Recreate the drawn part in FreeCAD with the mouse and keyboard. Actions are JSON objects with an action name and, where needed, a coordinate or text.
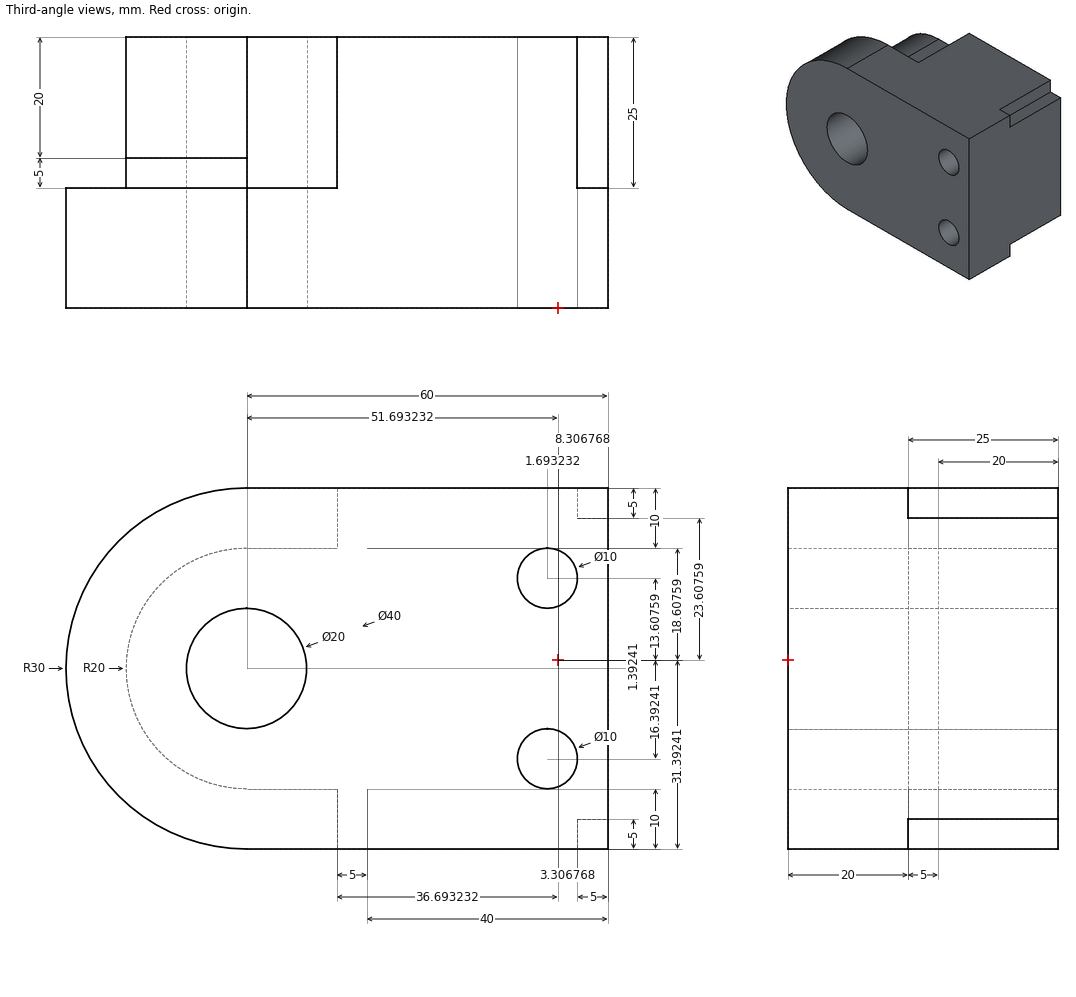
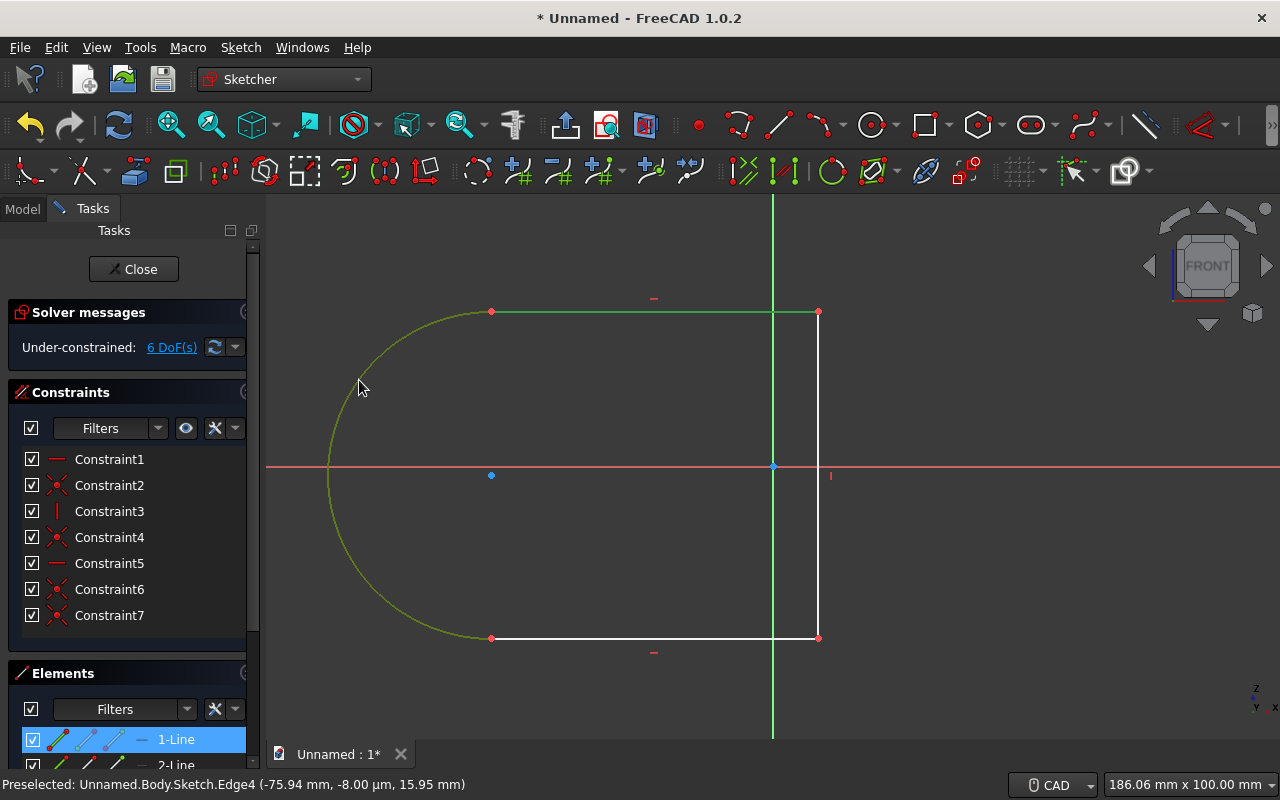
{"action": "key", "text": "t"}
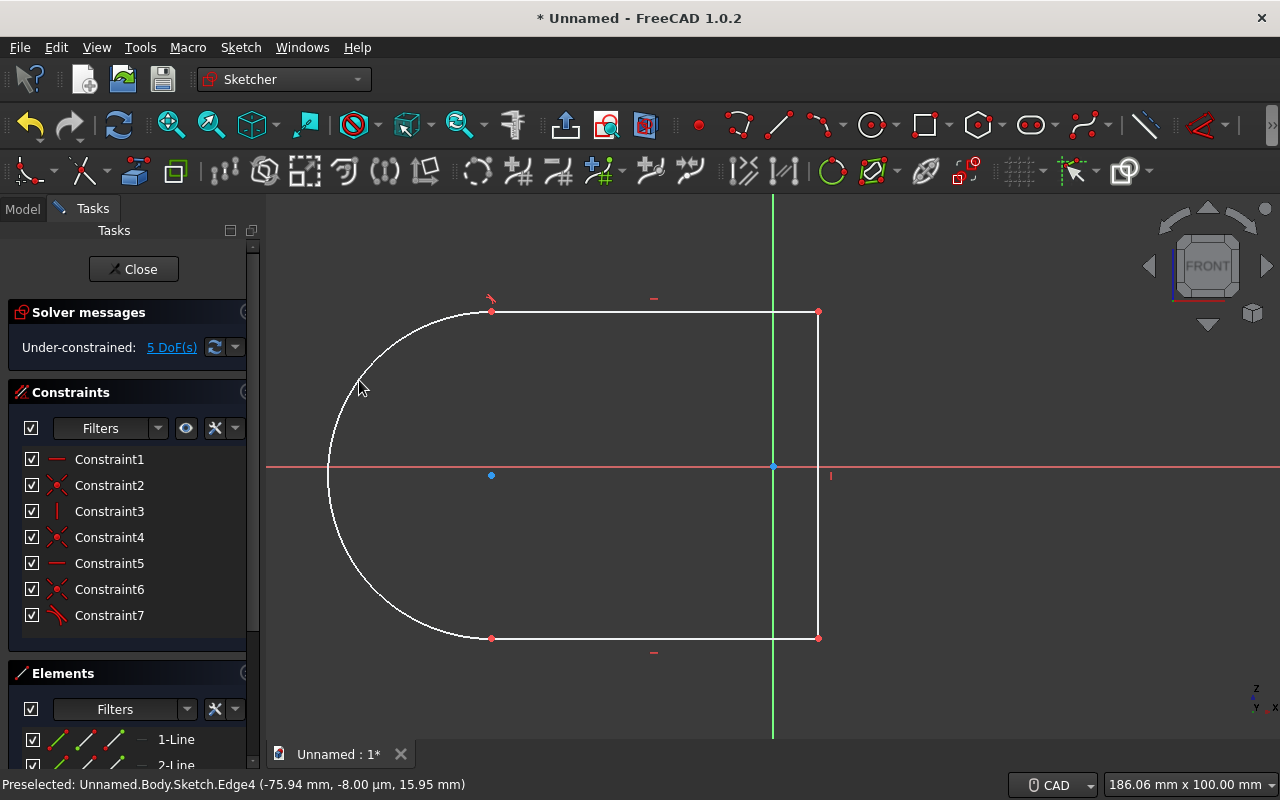
{"action": "left_click", "coordinate": [720, 639]}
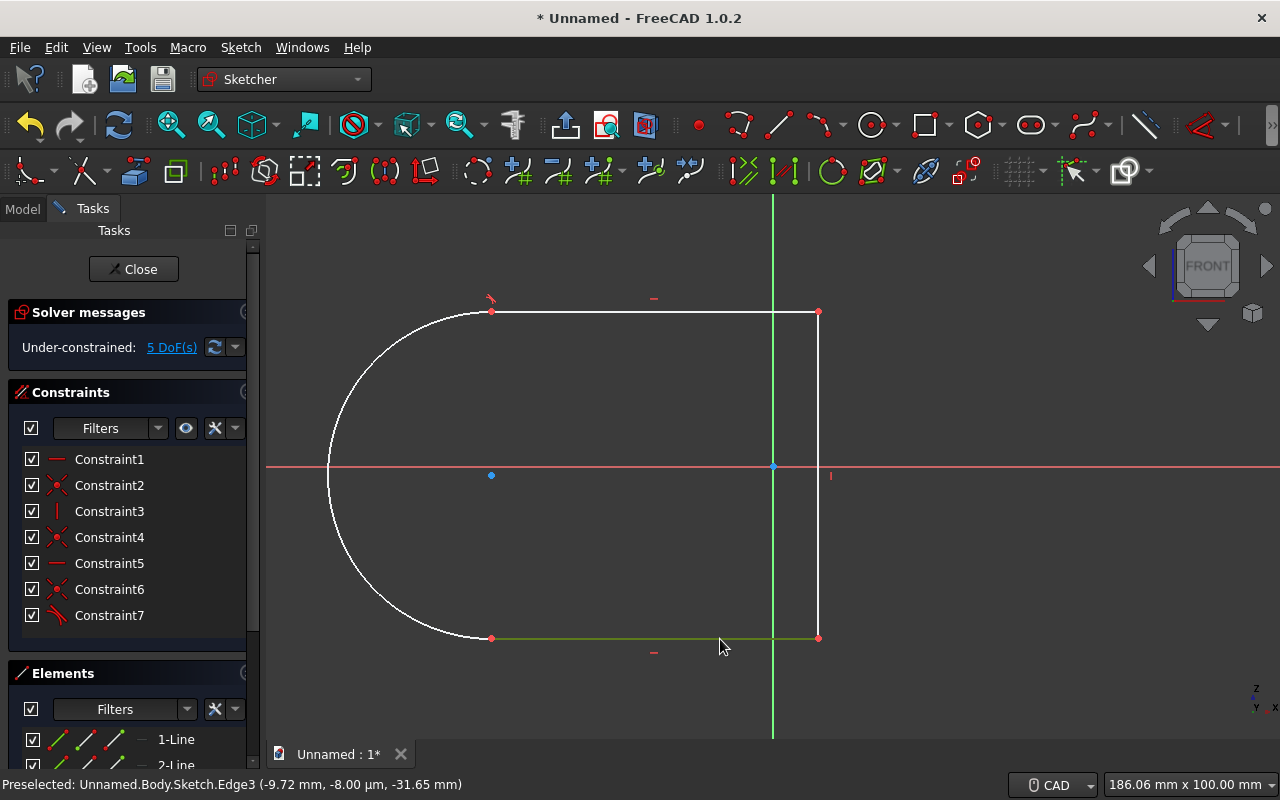
{"action": "left_click", "coordinate": [359, 379]}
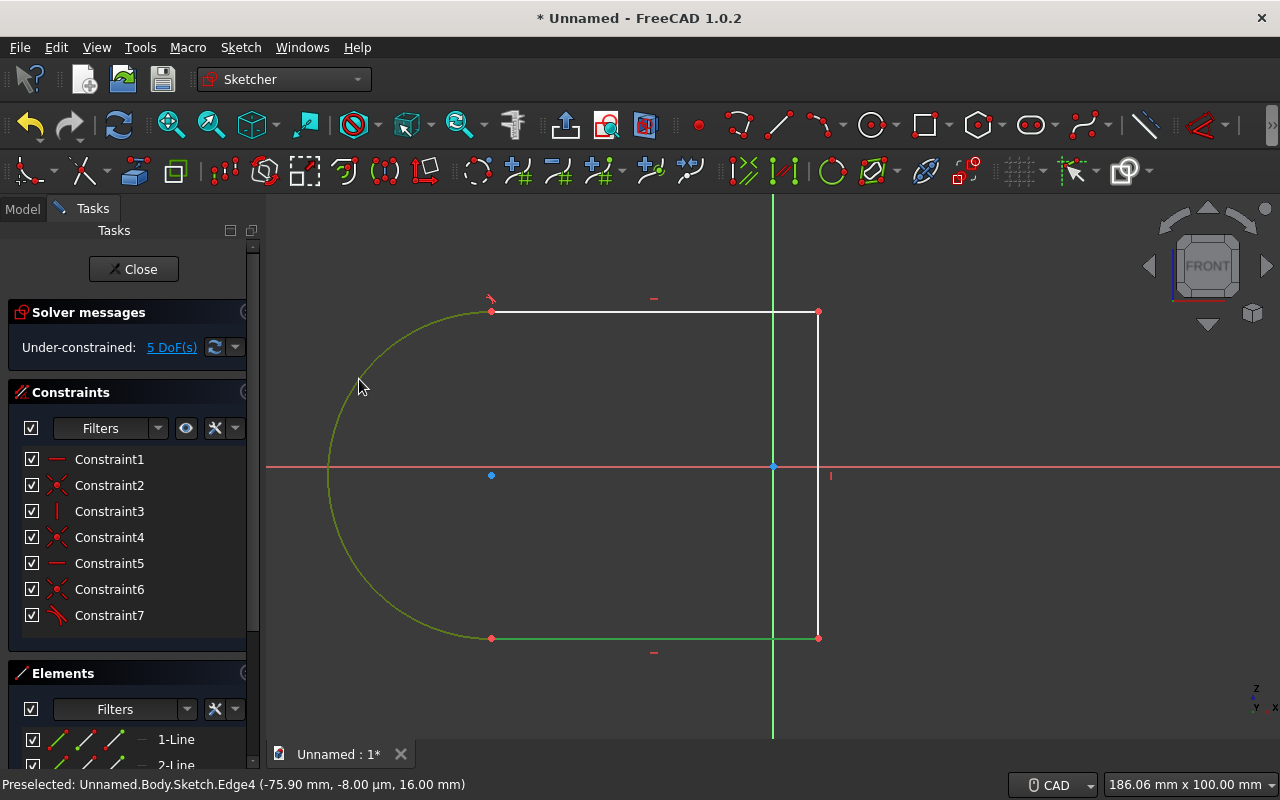
{"action": "key", "text": "t"}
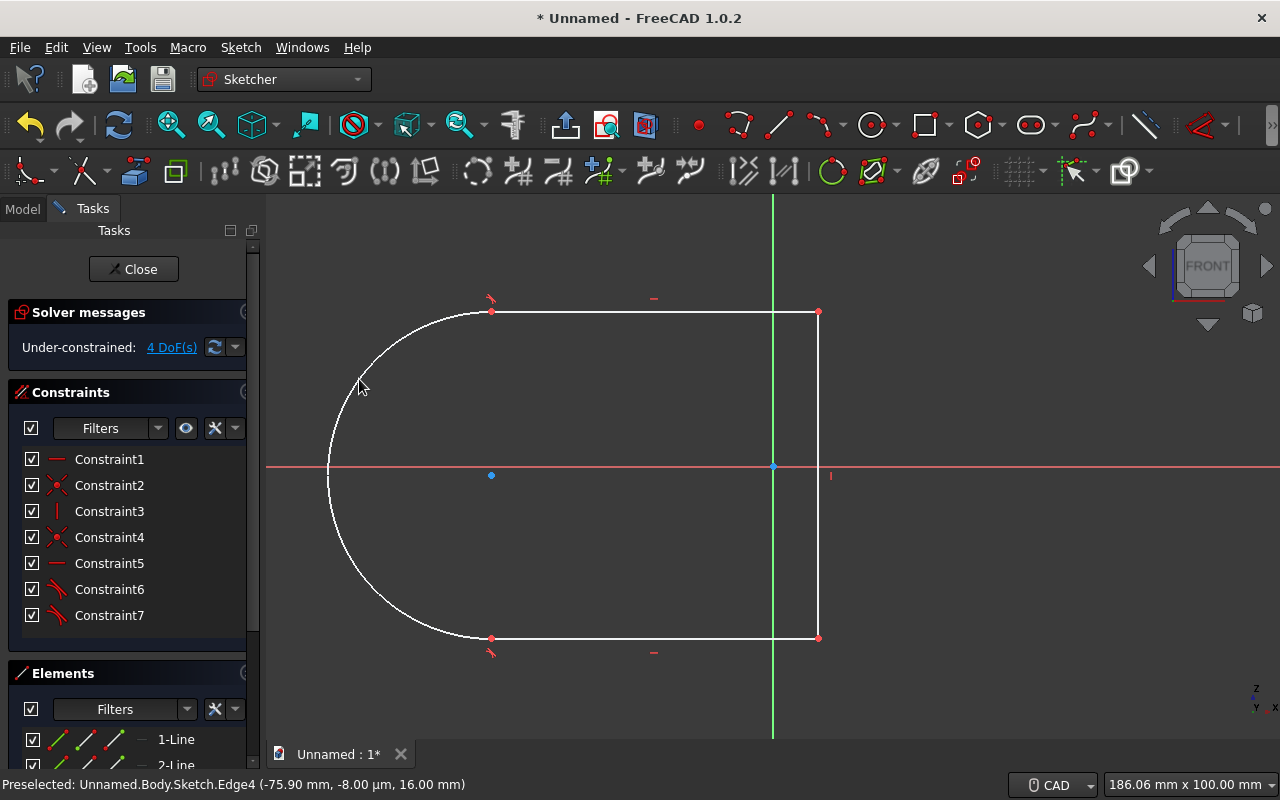
{"action": "key", "text": "d"}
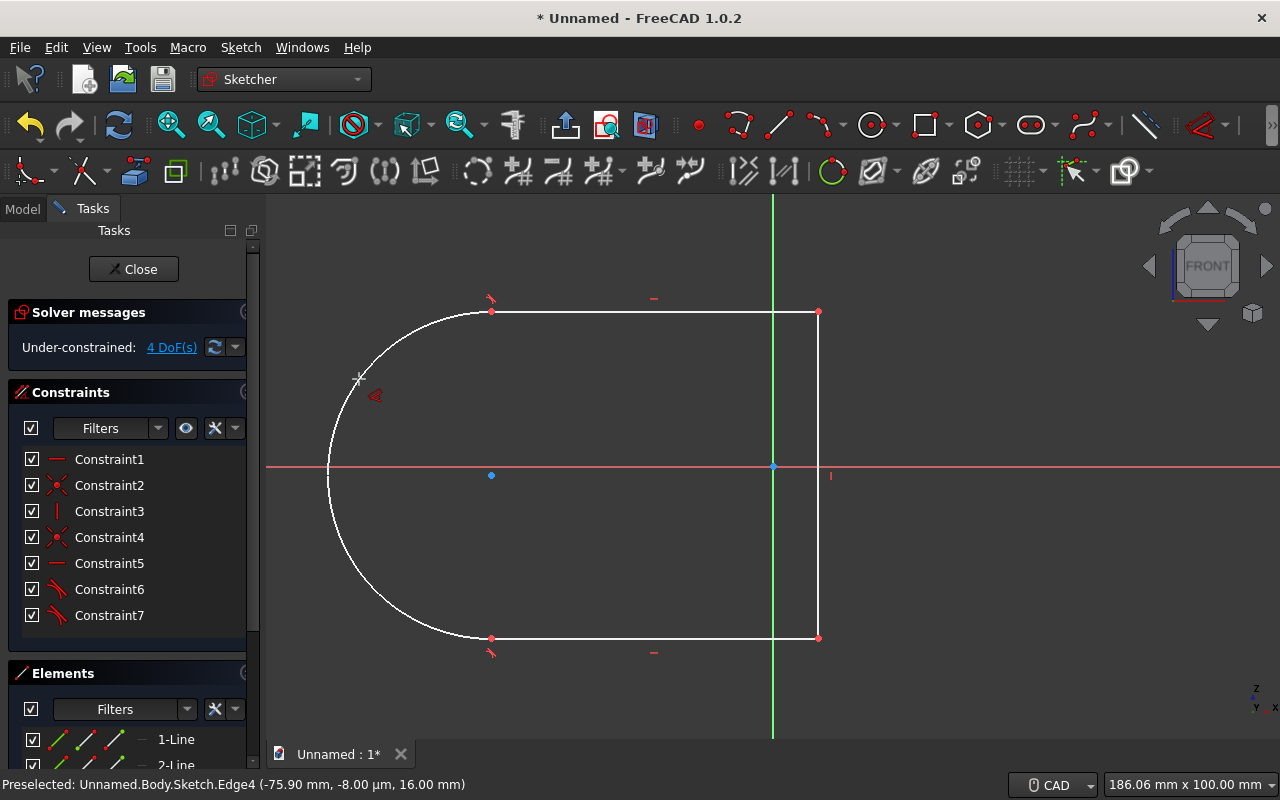
{"action": "left_click", "coordinate": [359, 379]}
{"action": "left_click", "coordinate": [333, 360]}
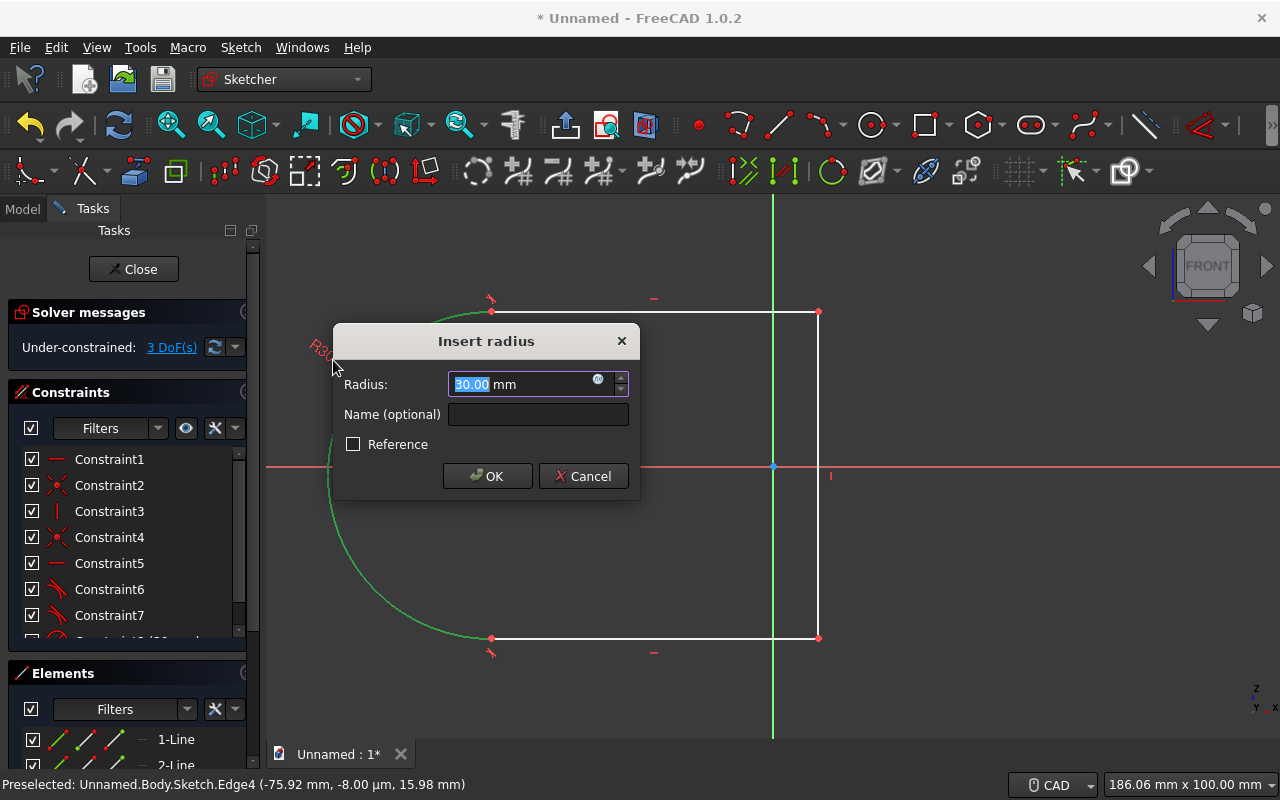
{"action": "type", "text": "30"}
{"action": "key", "text": "Return"}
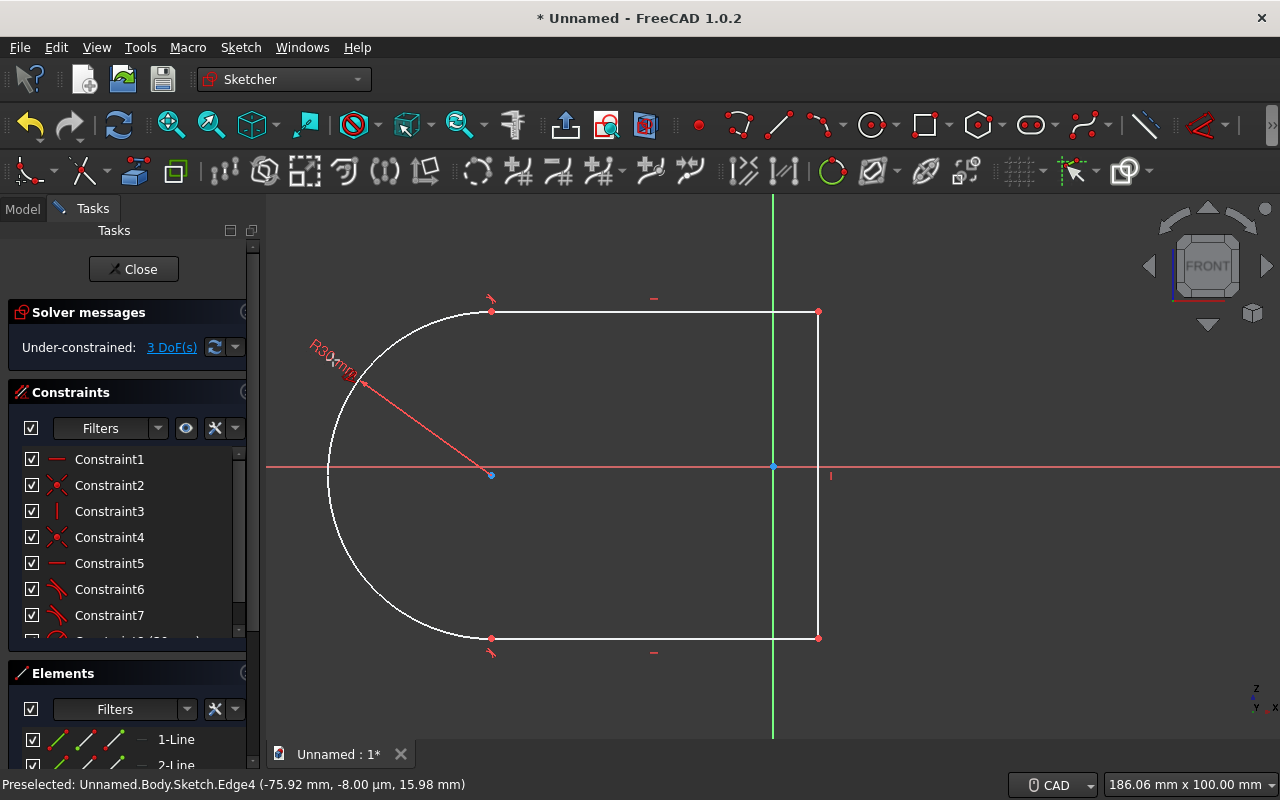
{"action": "left_click", "coordinate": [589, 312]}
{"action": "left_click", "coordinate": [655, 278]}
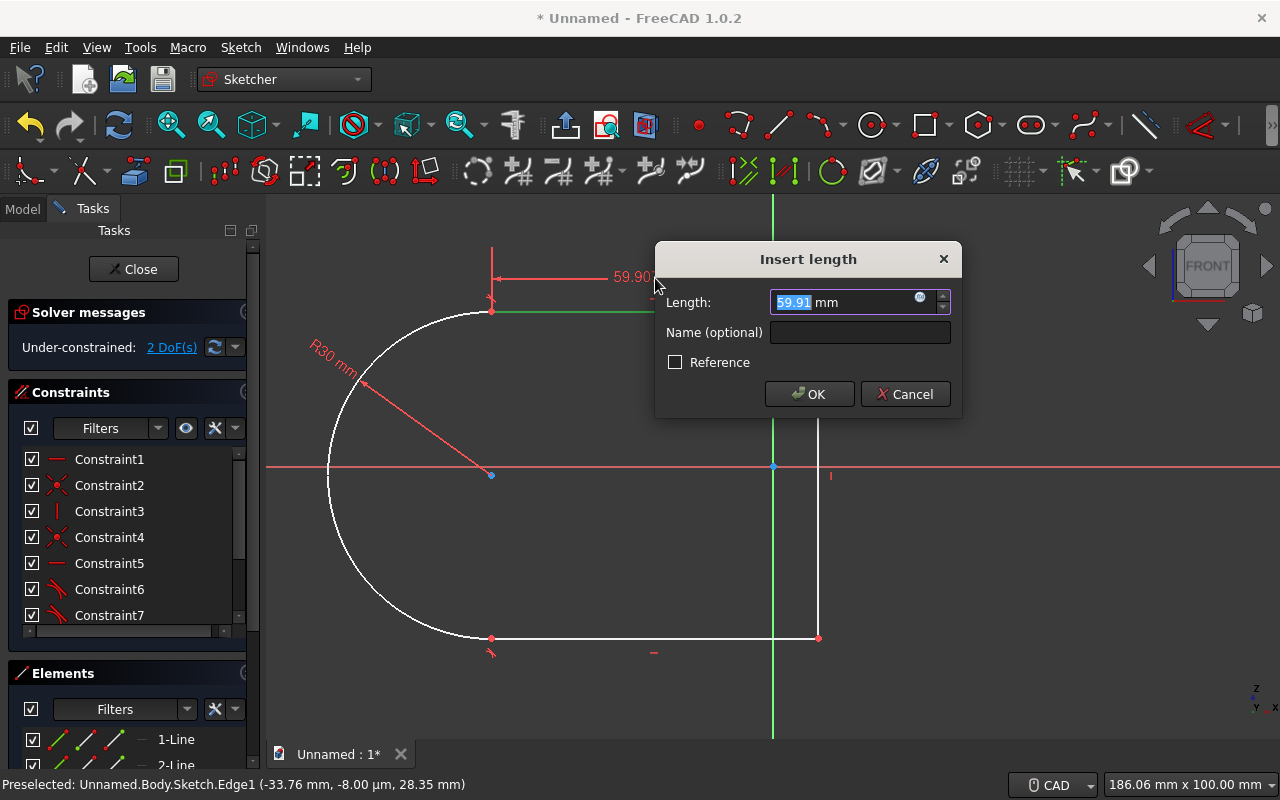
{"action": "type", "text": "60"}
{"action": "key", "text": "Return"}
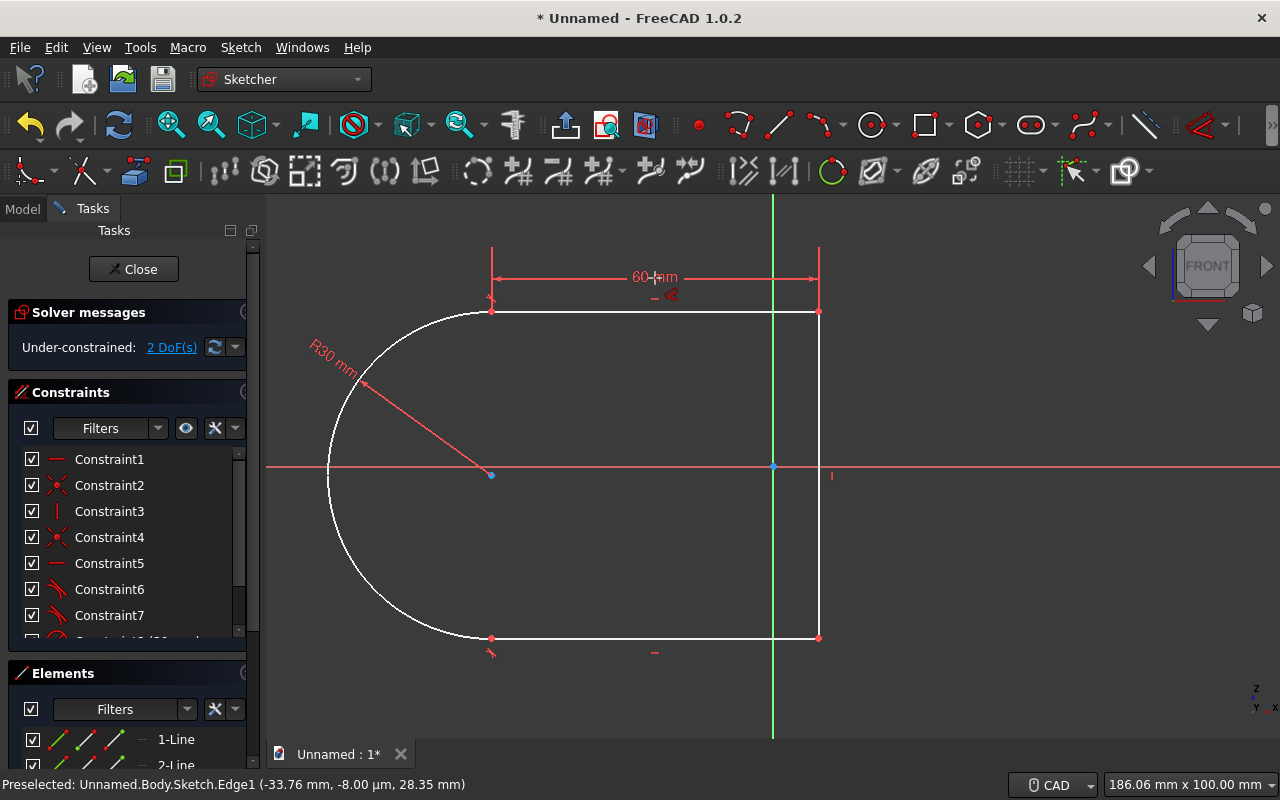
{"action": "scroll", "coordinate": [492, 475], "scroll_direction": "up", "scroll_amount": 9}